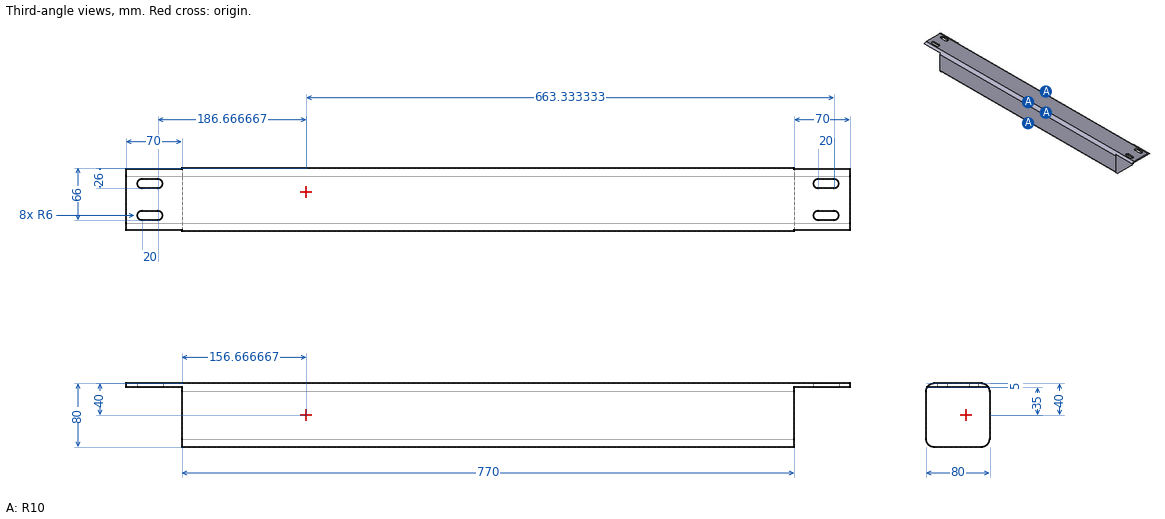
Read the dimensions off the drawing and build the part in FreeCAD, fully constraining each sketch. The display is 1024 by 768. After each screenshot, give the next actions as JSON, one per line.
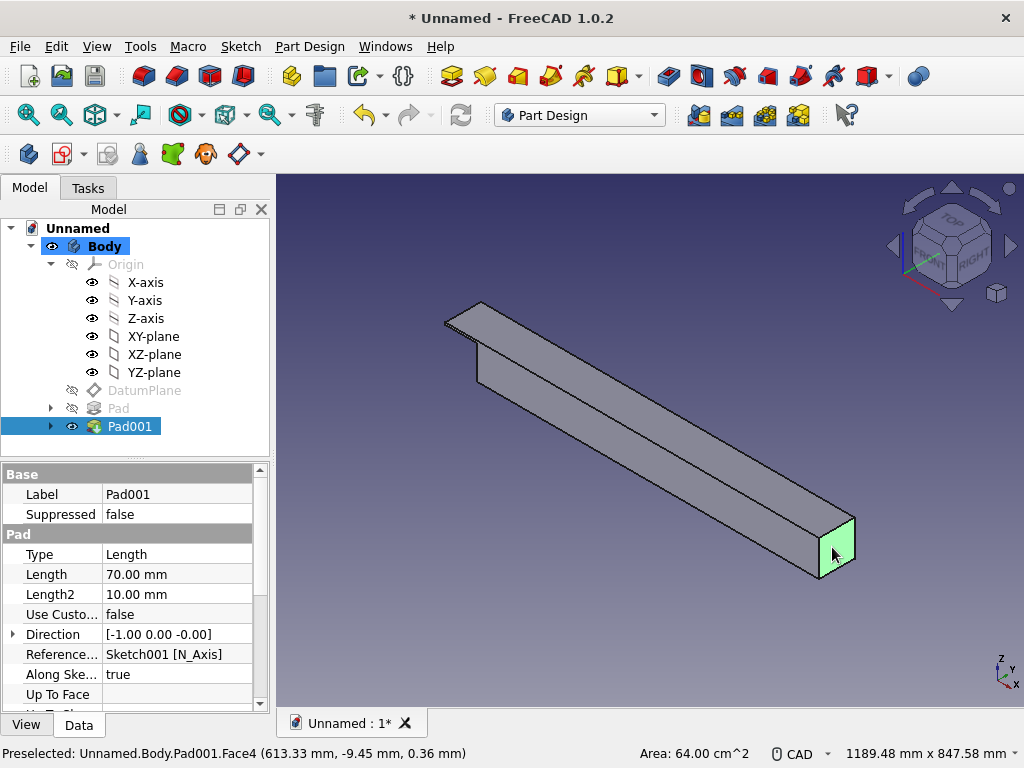
{"action": "left_click", "coordinate": [62, 154]}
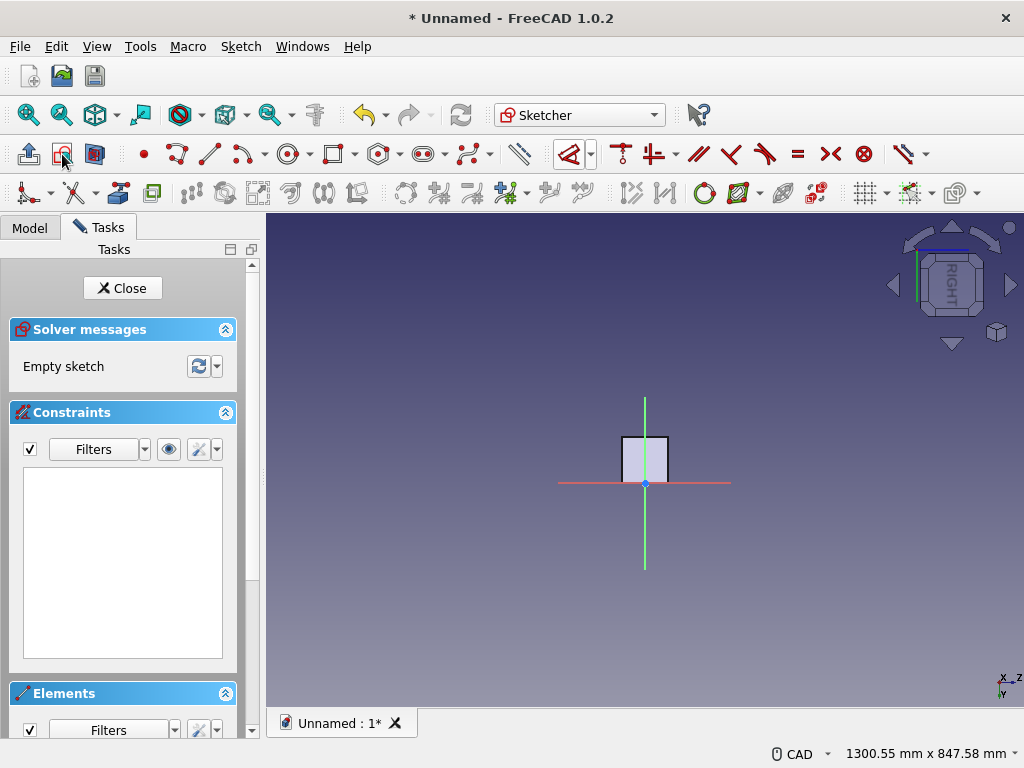
{"action": "scroll", "coordinate": [673, 460], "scroll_direction": "up", "scroll_amount": 9}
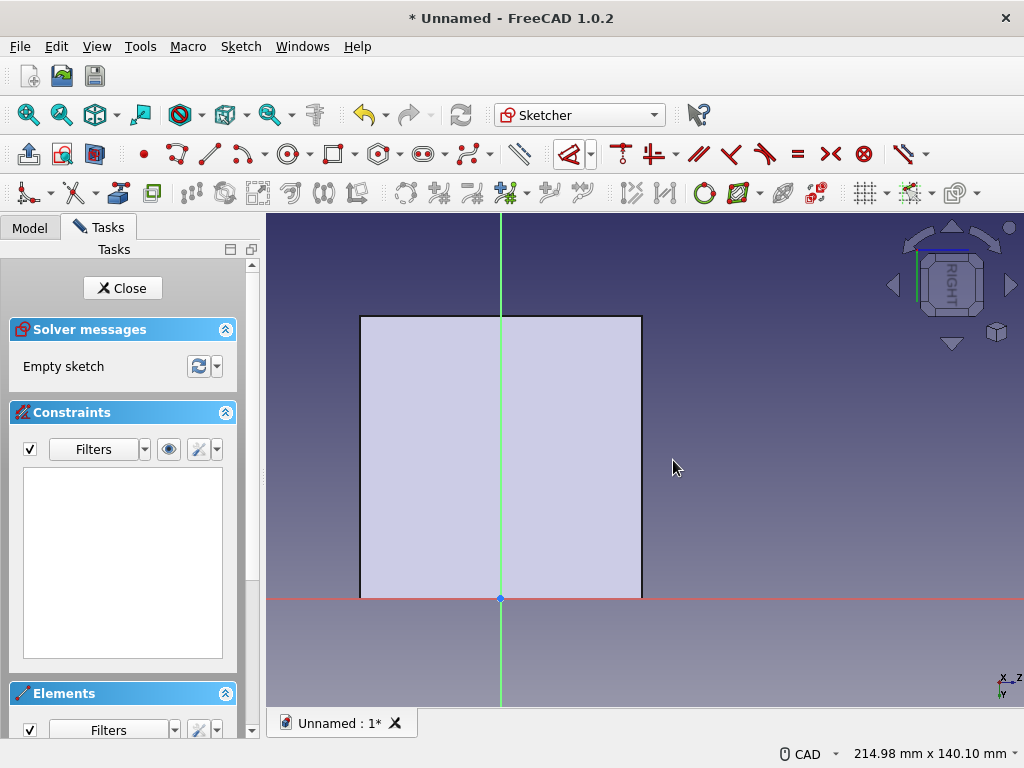
{"action": "left_click", "coordinate": [332, 154]}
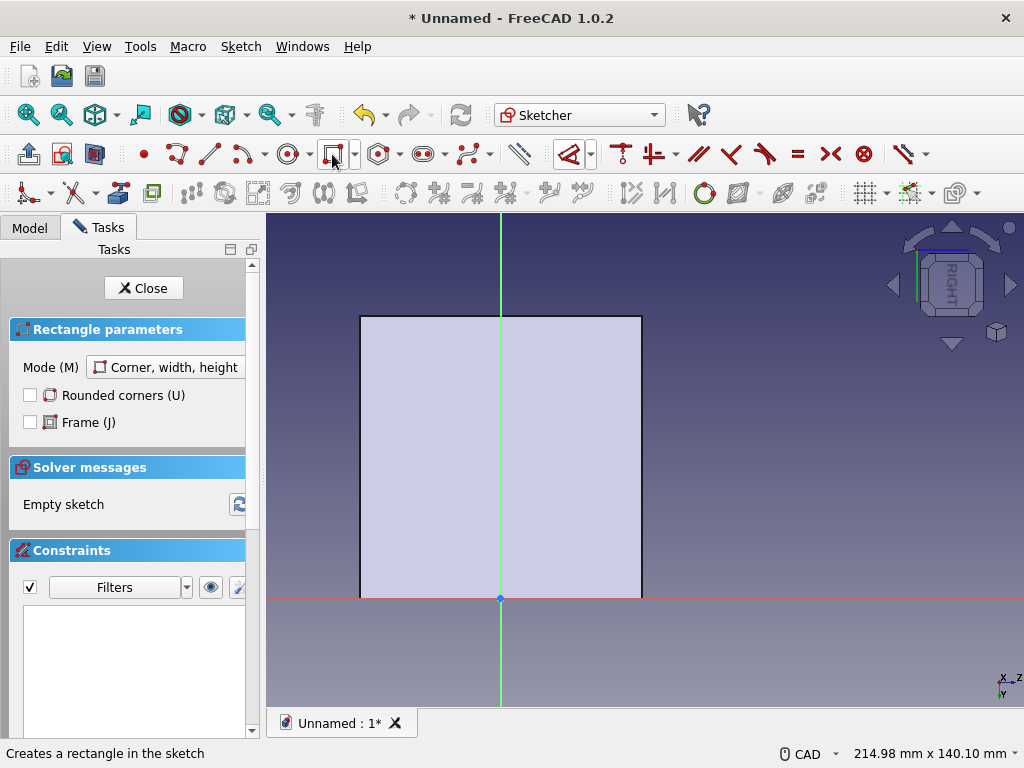
{"action": "left_click", "coordinate": [624, 316]}
{"action": "left_click", "coordinate": [642, 599]}
{"action": "key", "text": "Escape"}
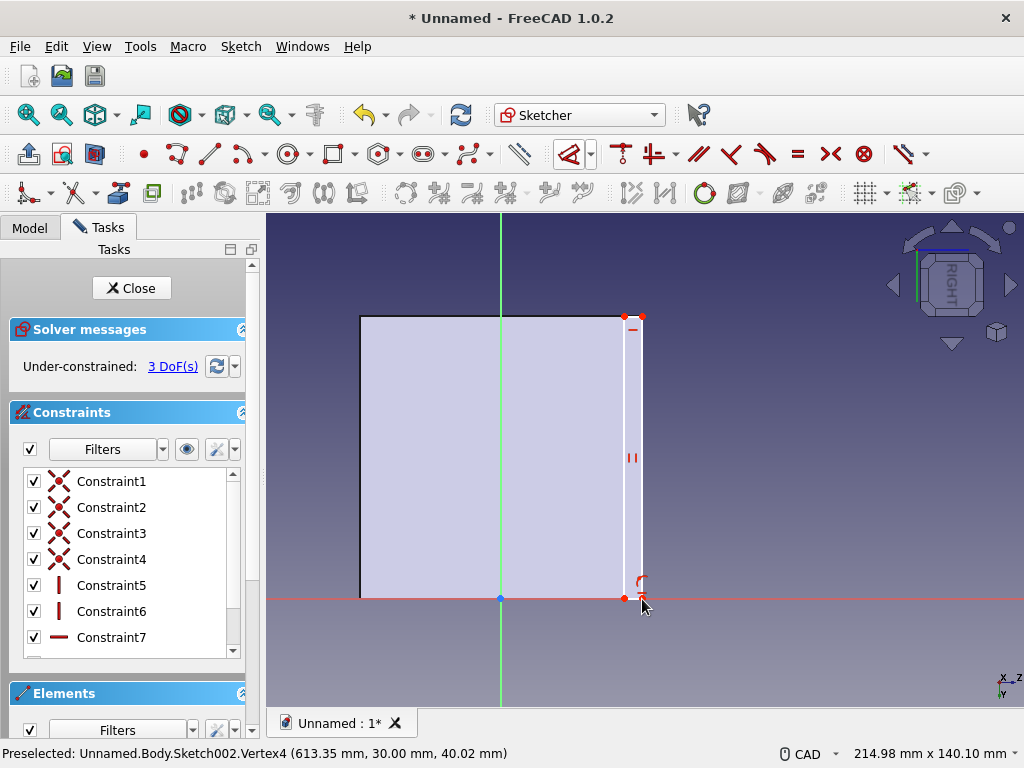
{"action": "scroll", "coordinate": [633, 599], "scroll_direction": "up", "scroll_amount": 5}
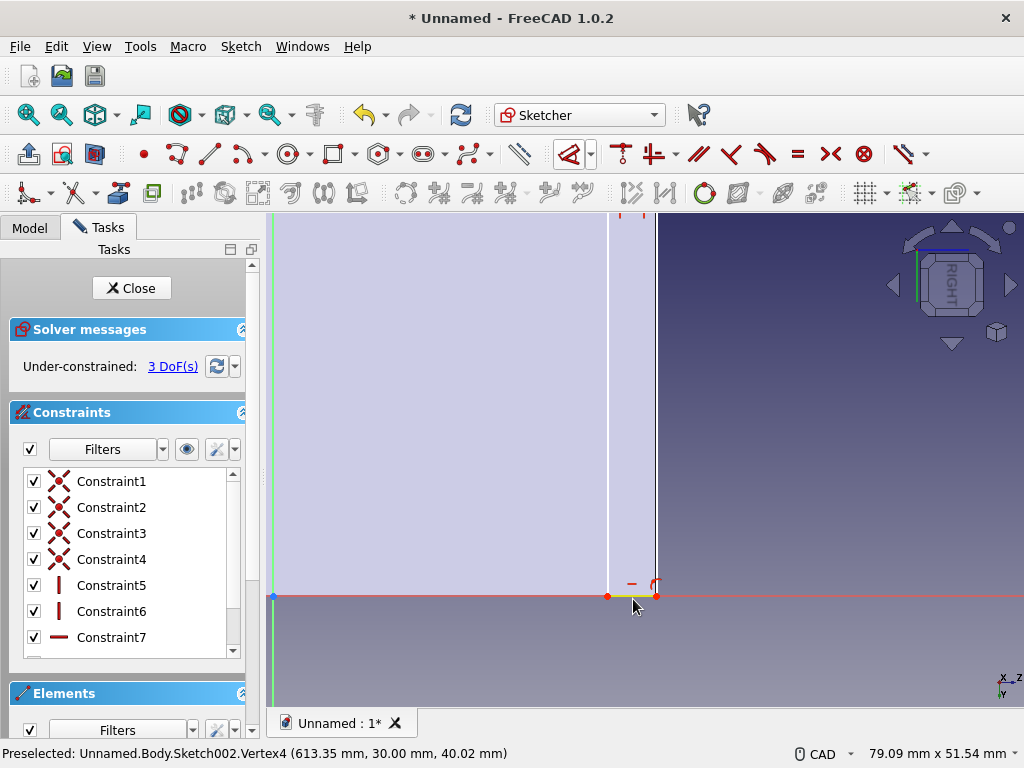
{"action": "left_click", "coordinate": [632, 596]}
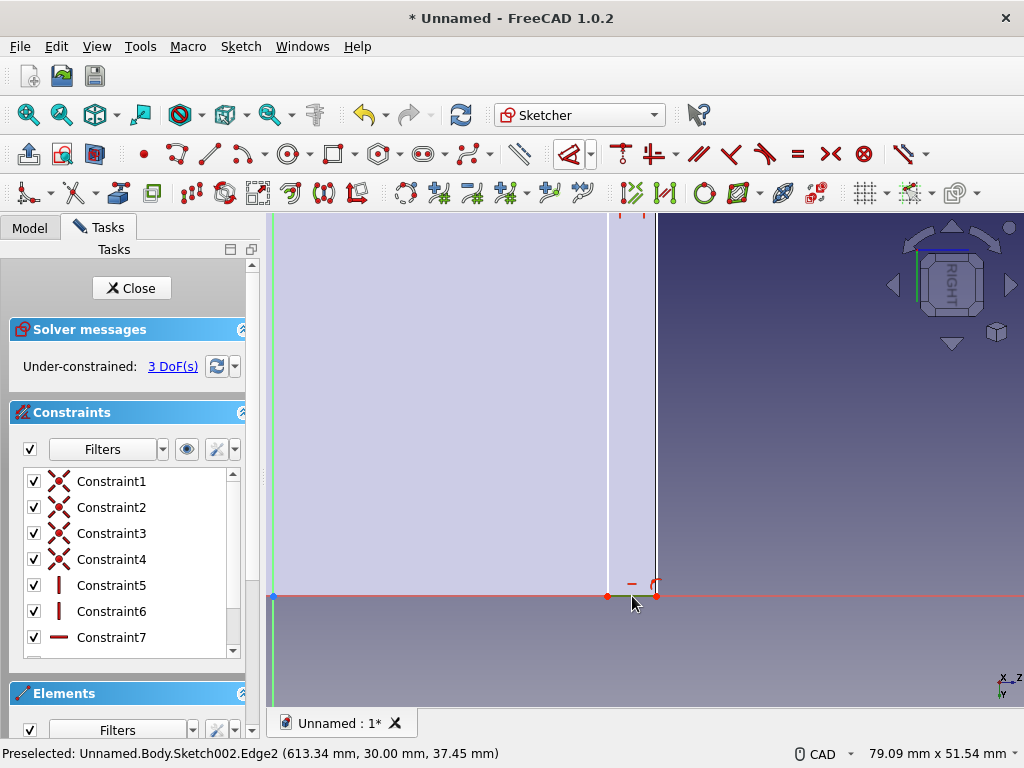
{"action": "left_click", "coordinate": [590, 154]}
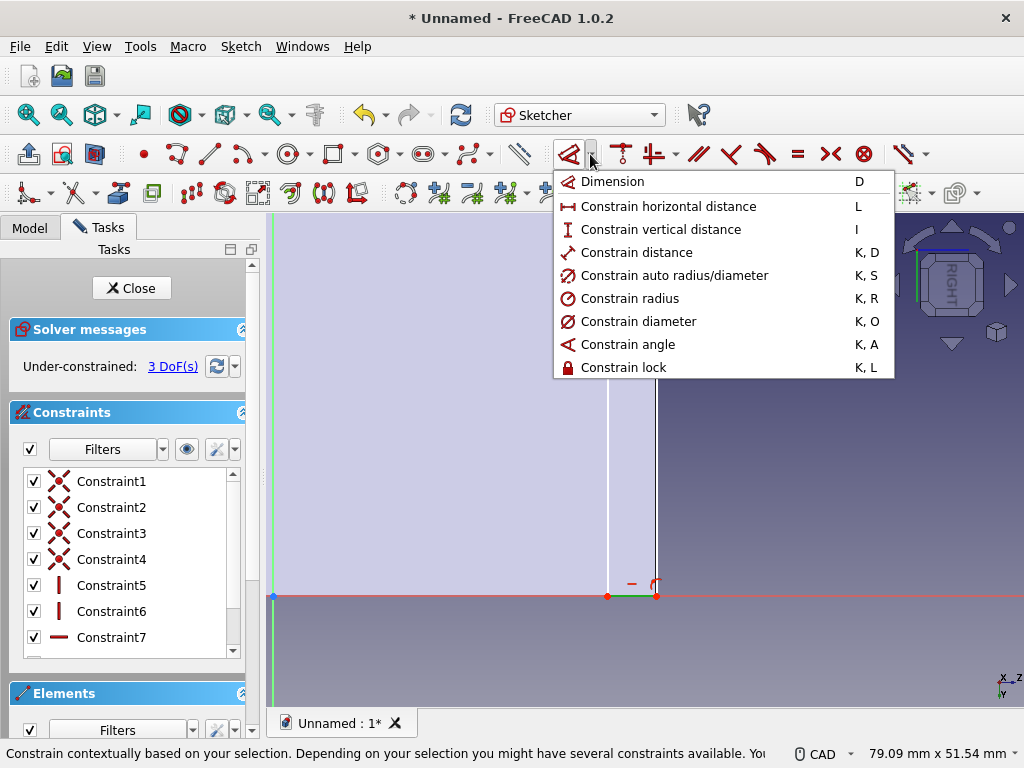
{"action": "left_click", "coordinate": [724, 206]}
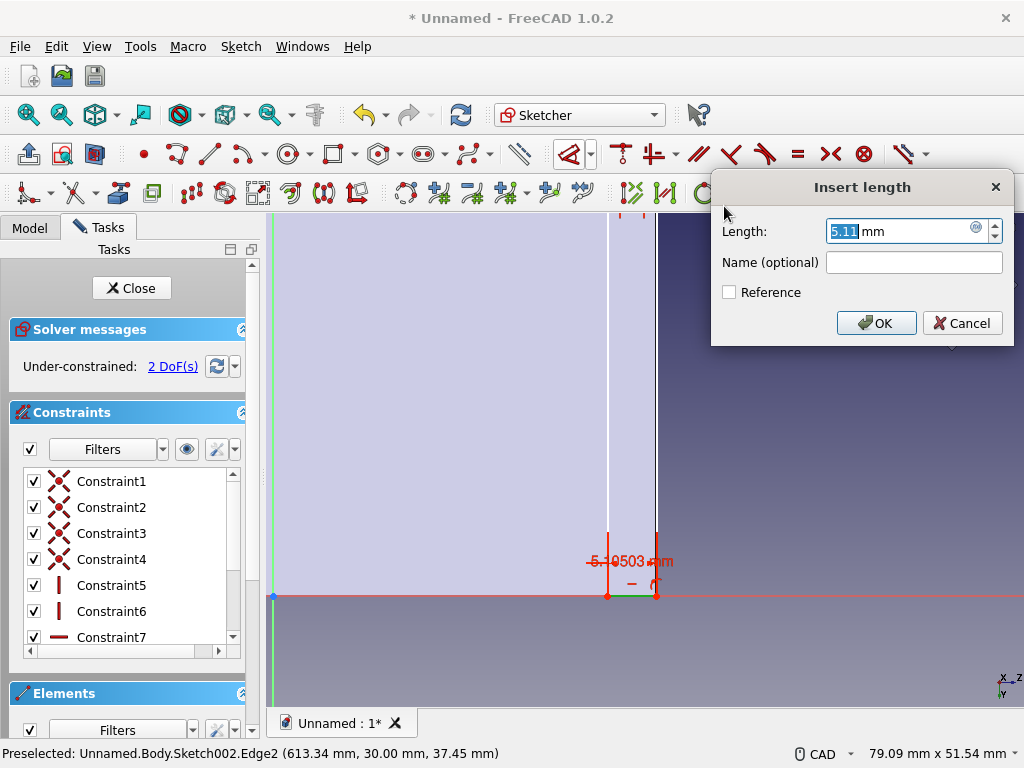
{"action": "type", "text": "5"}
{"action": "key", "text": "Return"}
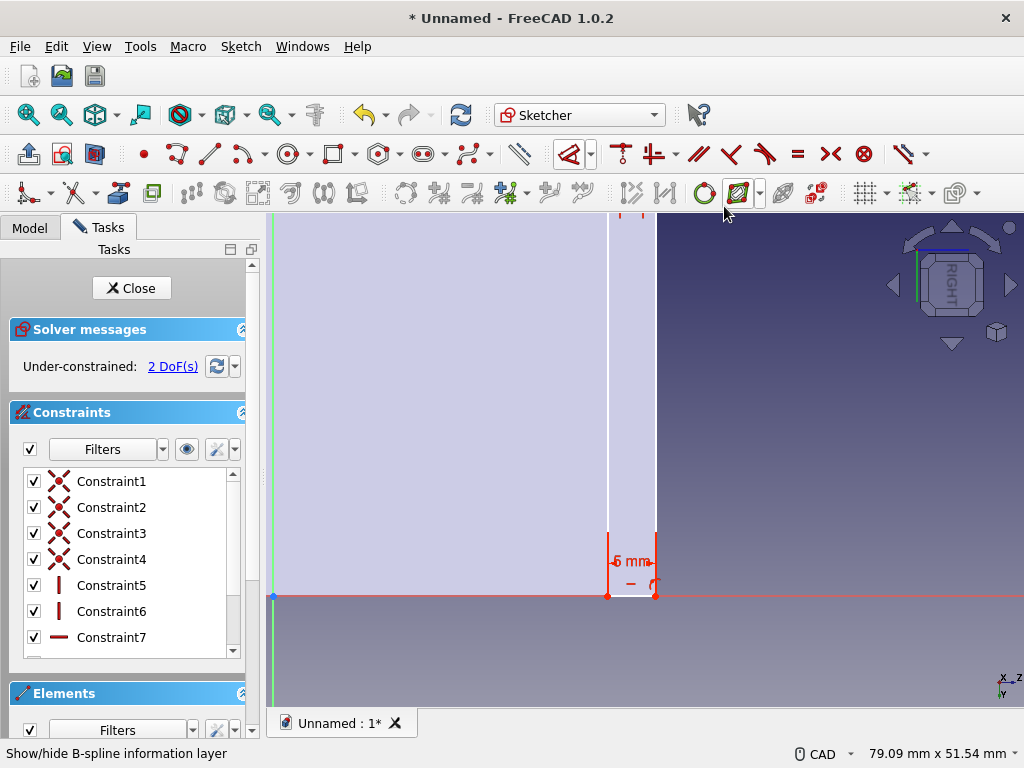
{"action": "left_click", "coordinate": [608, 367]}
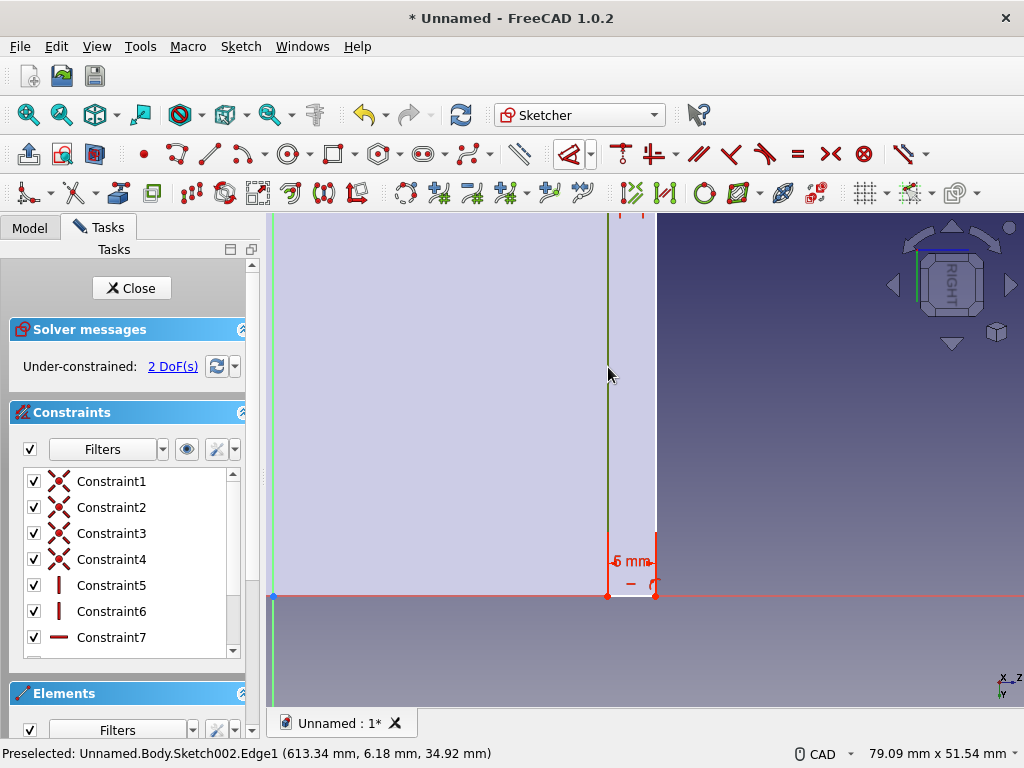
{"action": "left_click", "coordinate": [590, 154]}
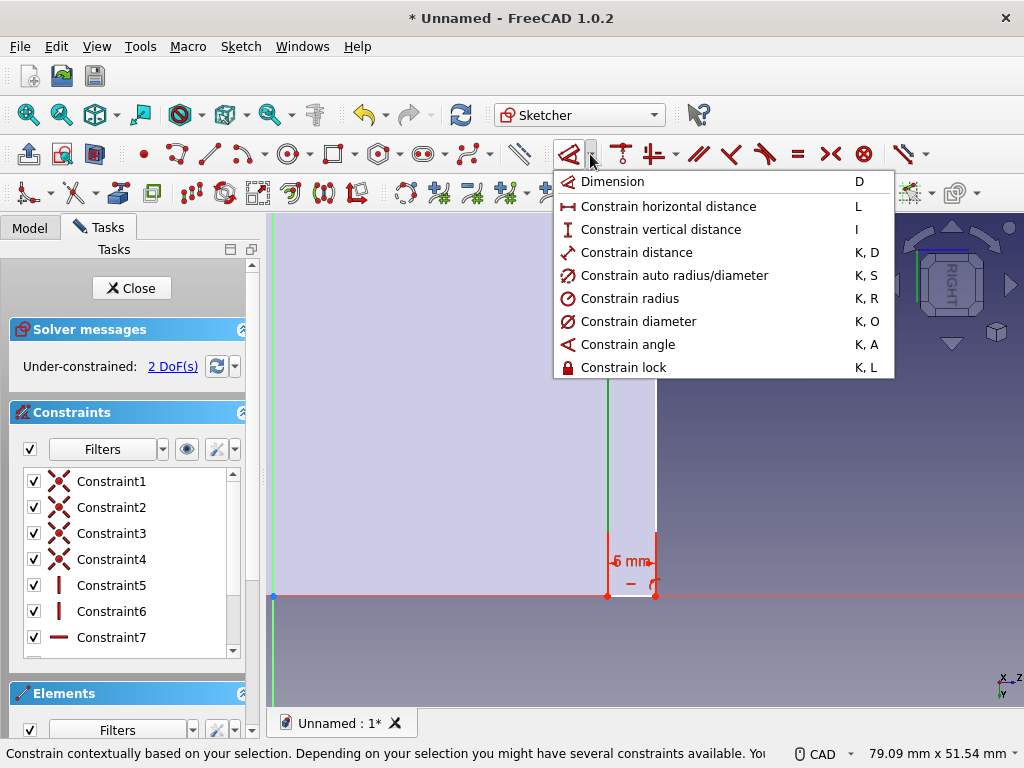
{"action": "left_click", "coordinate": [724, 230]}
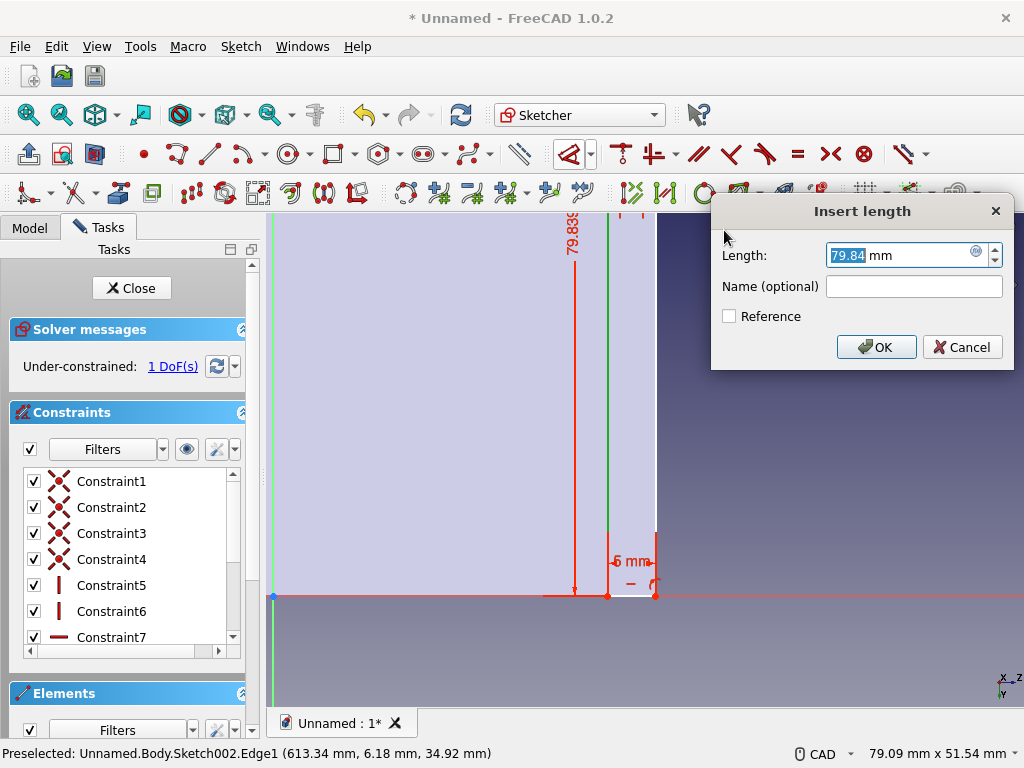
{"action": "type", "text": "80"}
{"action": "key", "text": "Return"}